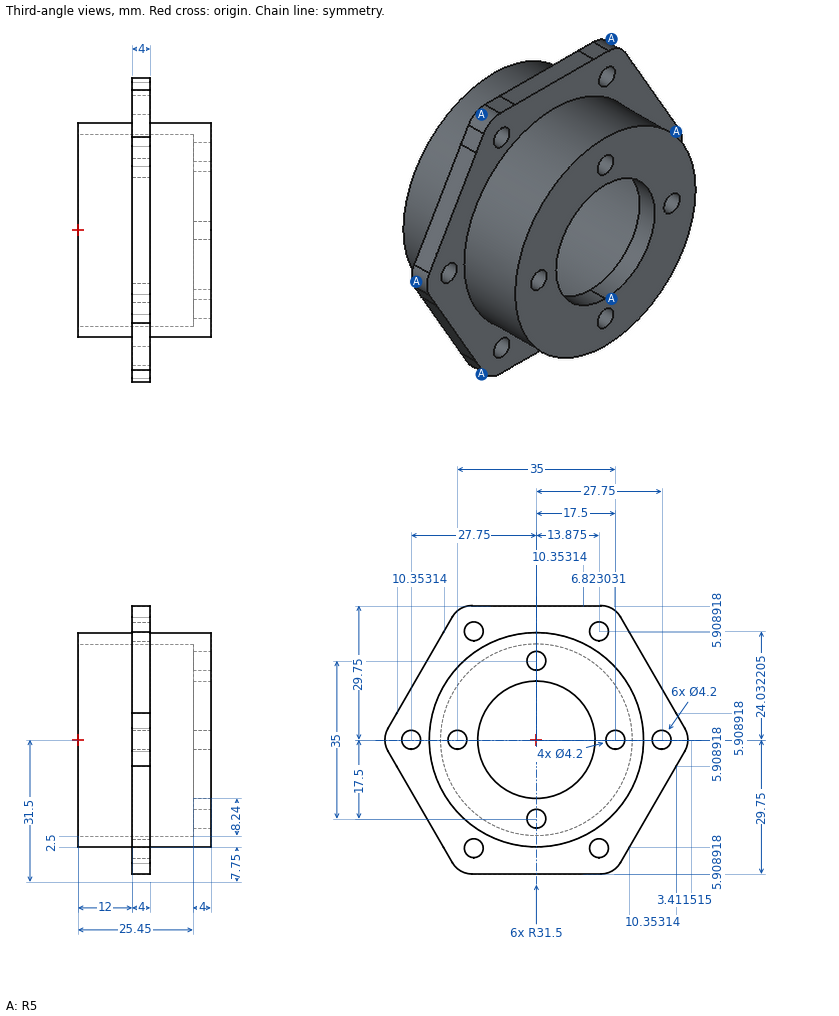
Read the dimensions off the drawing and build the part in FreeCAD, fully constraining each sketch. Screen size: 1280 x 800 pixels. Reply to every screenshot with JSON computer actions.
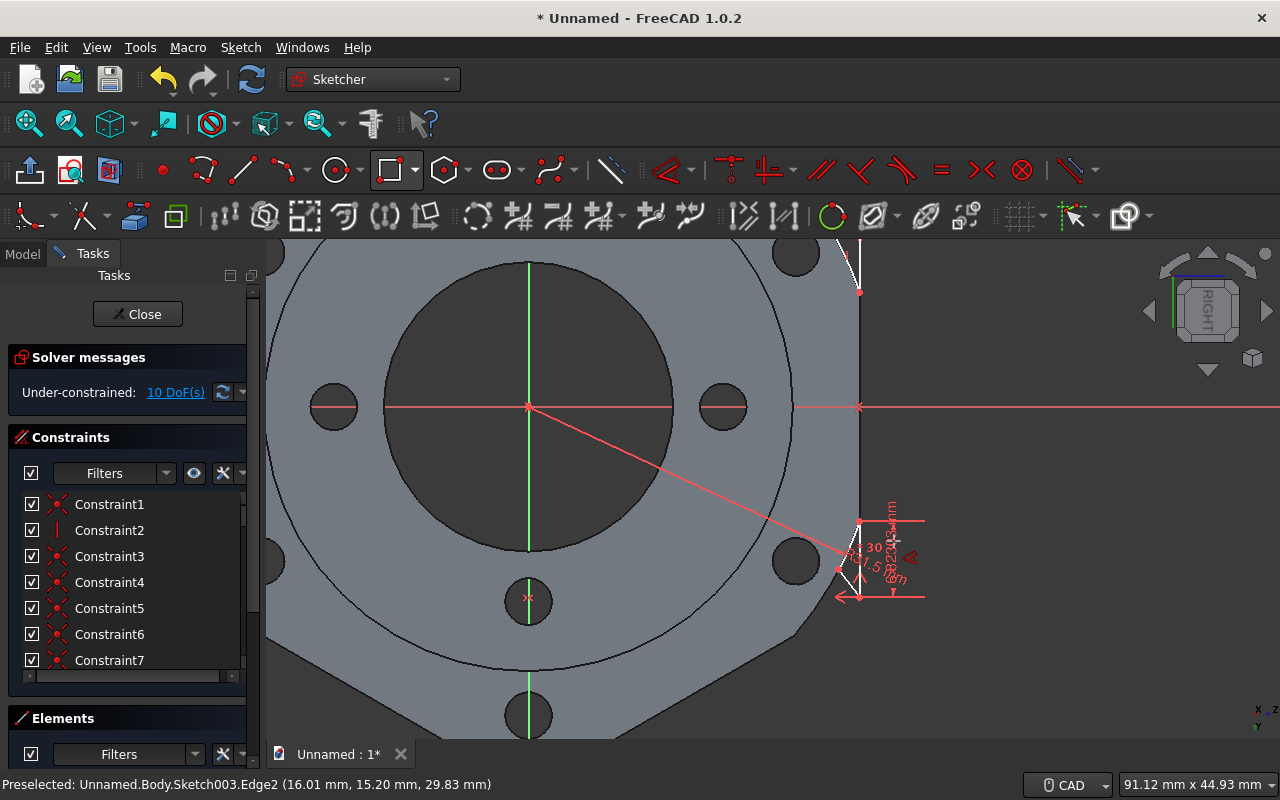
{"action": "left_click", "coordinate": [860, 521]}
{"action": "left_click", "coordinate": [894, 464]}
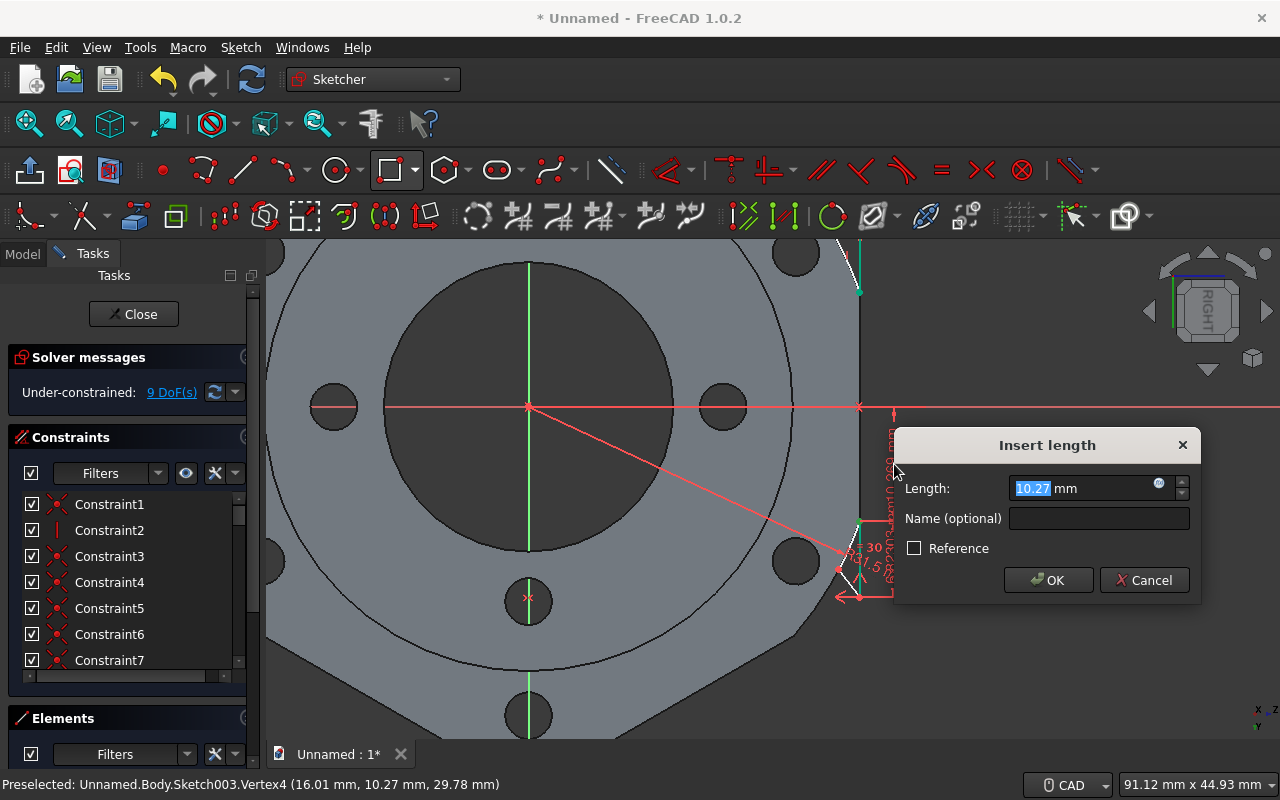
{"action": "type", "text": "10.35314"}
{"action": "key", "text": "Return"}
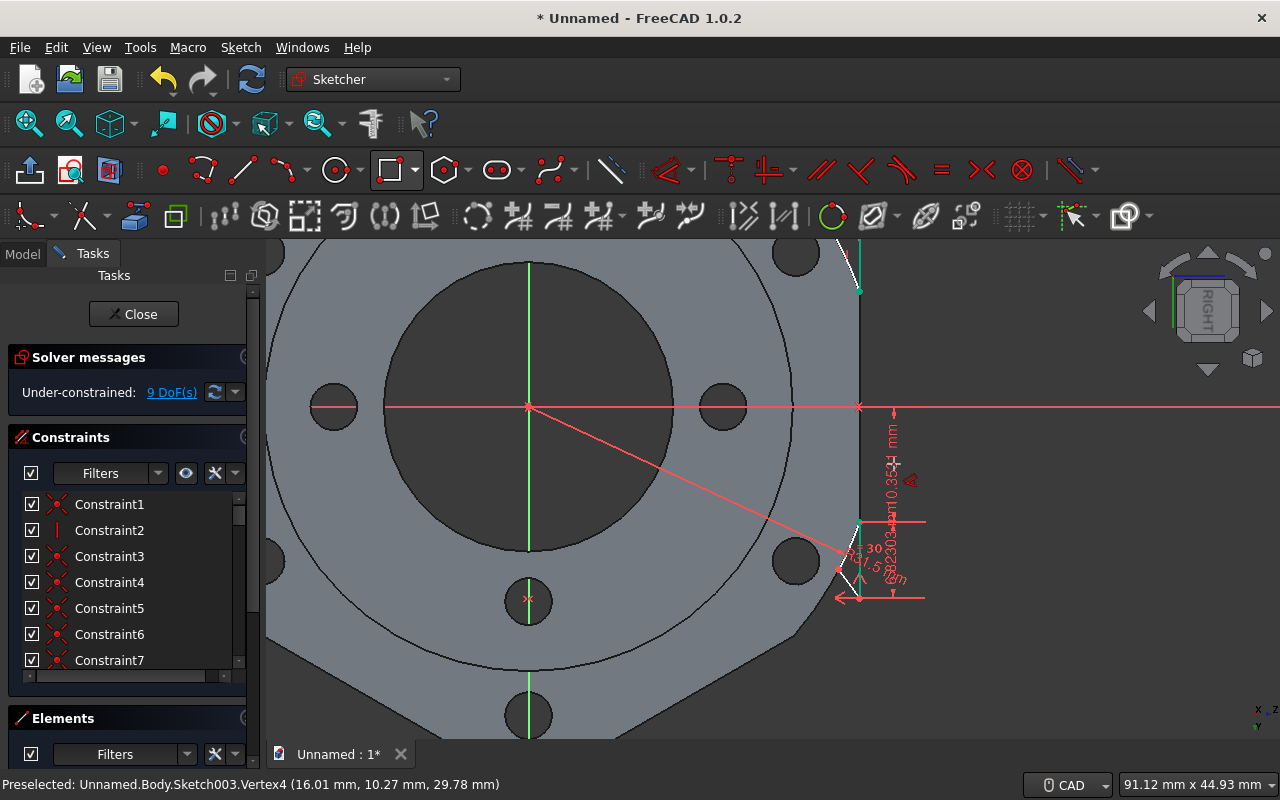
{"action": "scroll", "coordinate": [848, 556], "scroll_direction": "down", "scroll_amount": 4}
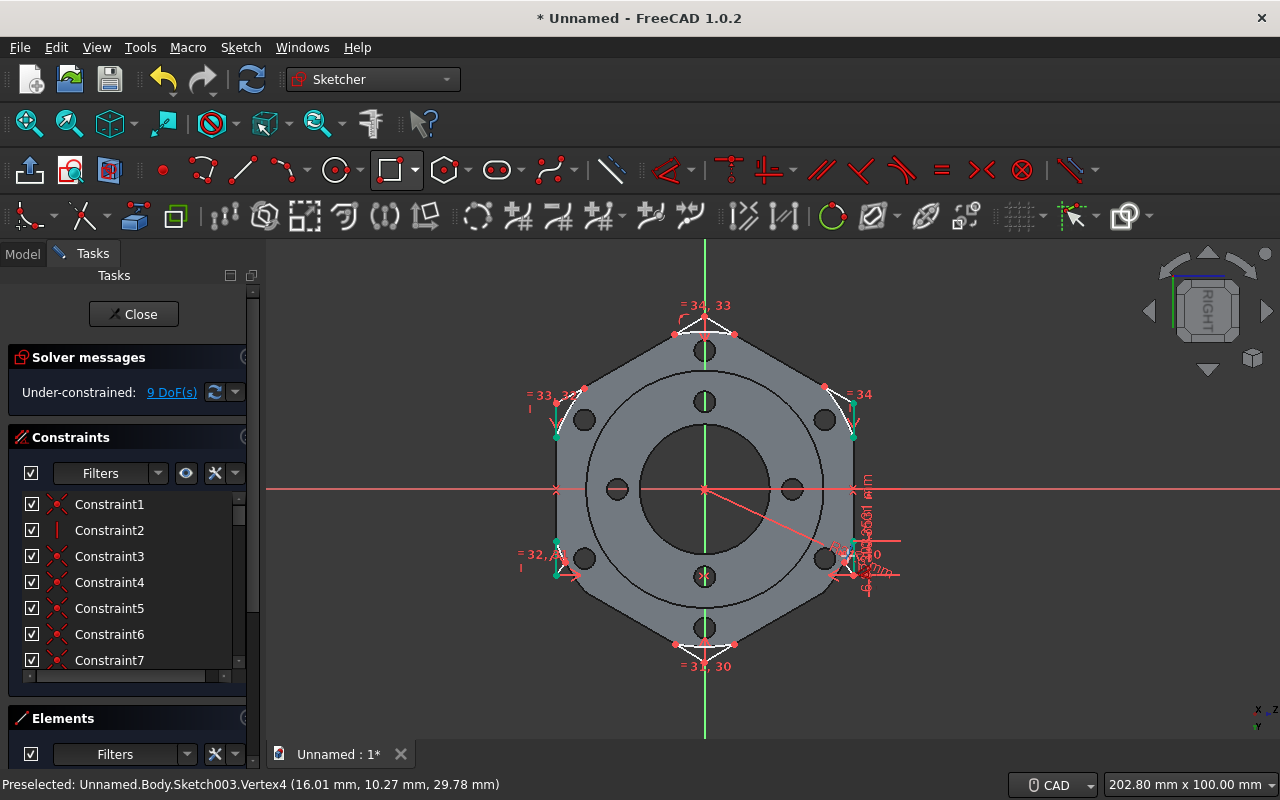
{"action": "scroll", "coordinate": [675, 644], "scroll_direction": "up", "scroll_amount": 2}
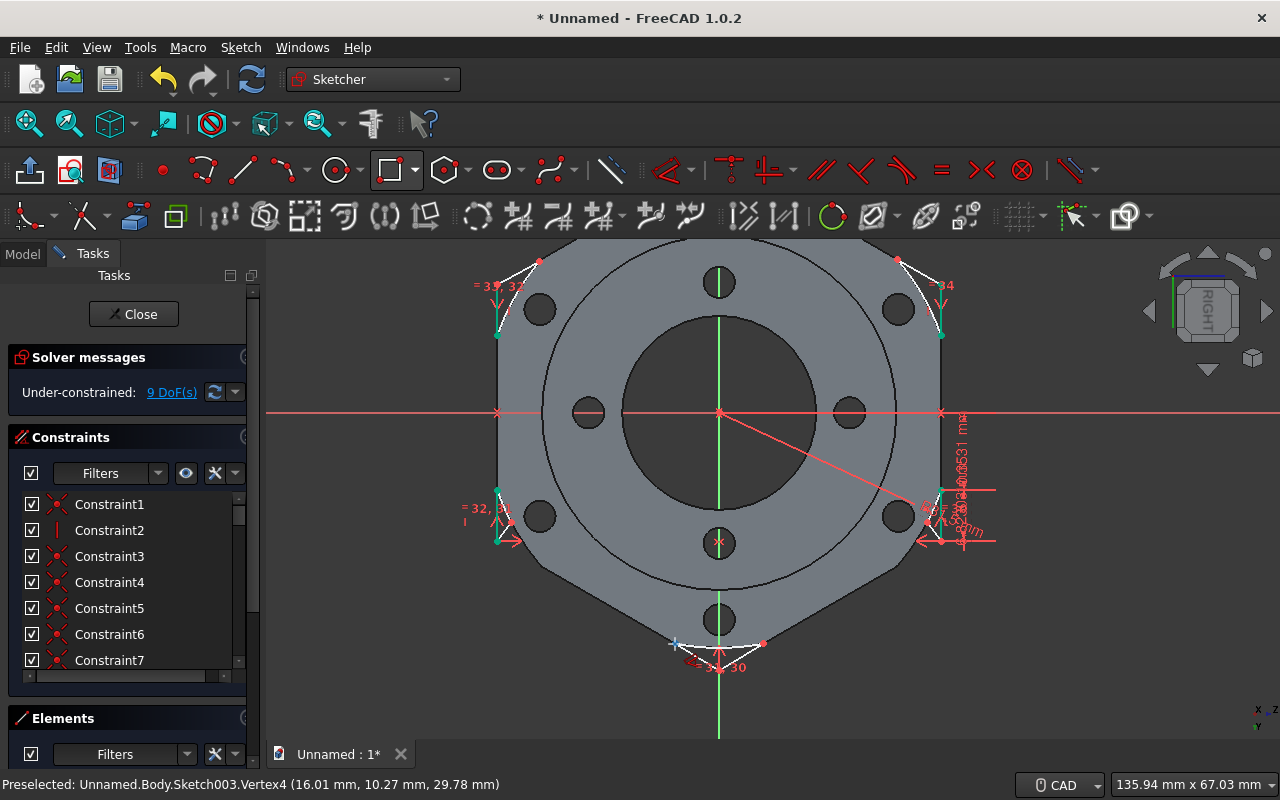
{"action": "left_click", "coordinate": [675, 644]}
{"action": "left_click", "coordinate": [697, 678]}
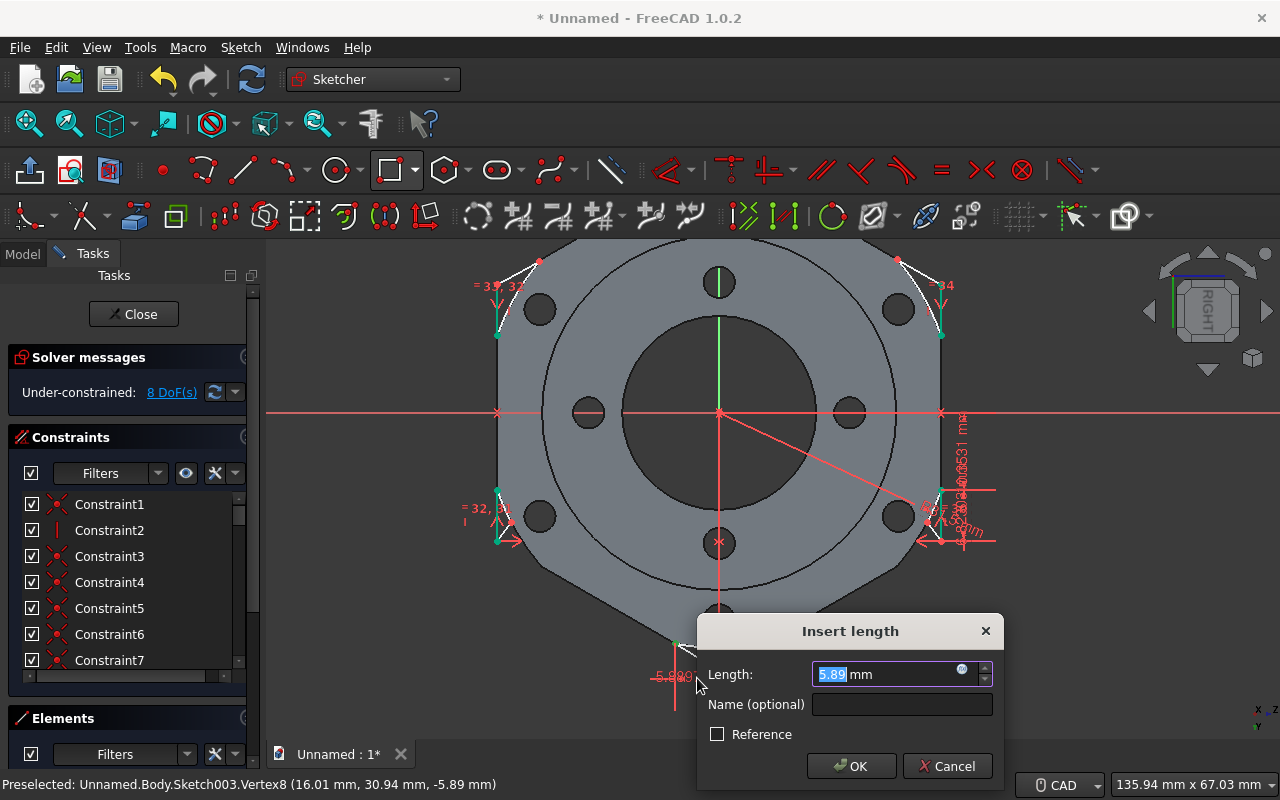
{"action": "type", "text": "5.908918"}
{"action": "key", "text": "Return"}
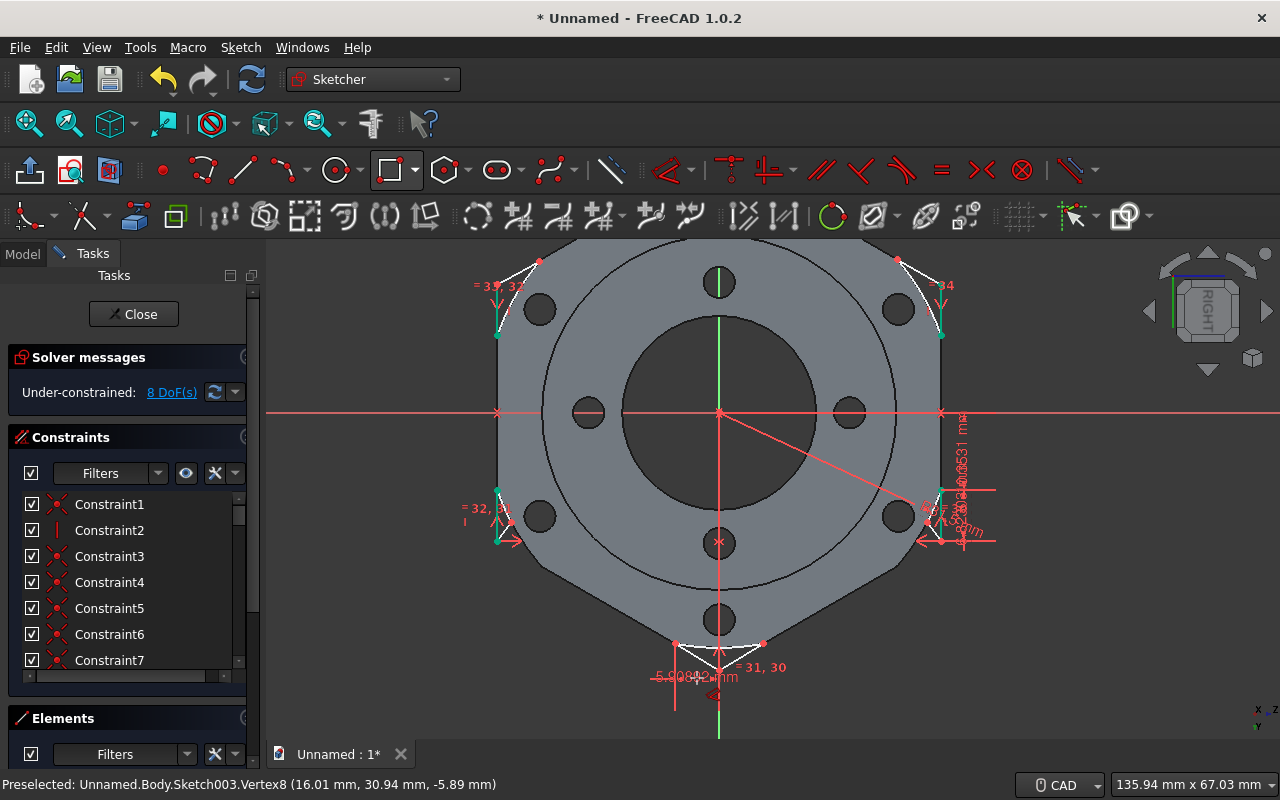
{"action": "left_click", "coordinate": [764, 644]}
{"action": "left_click", "coordinate": [741, 379]}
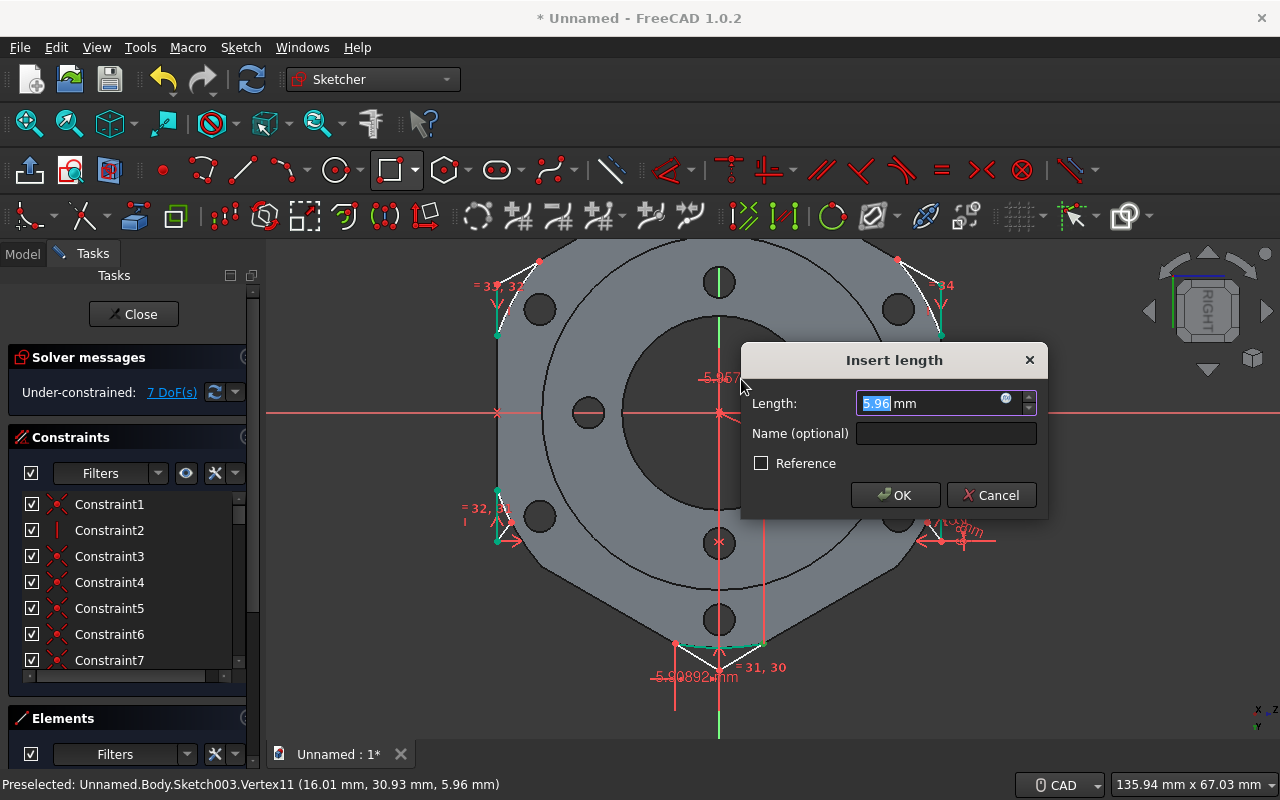
{"action": "type", "text": "5.908918"}
{"action": "key", "text": "Return"}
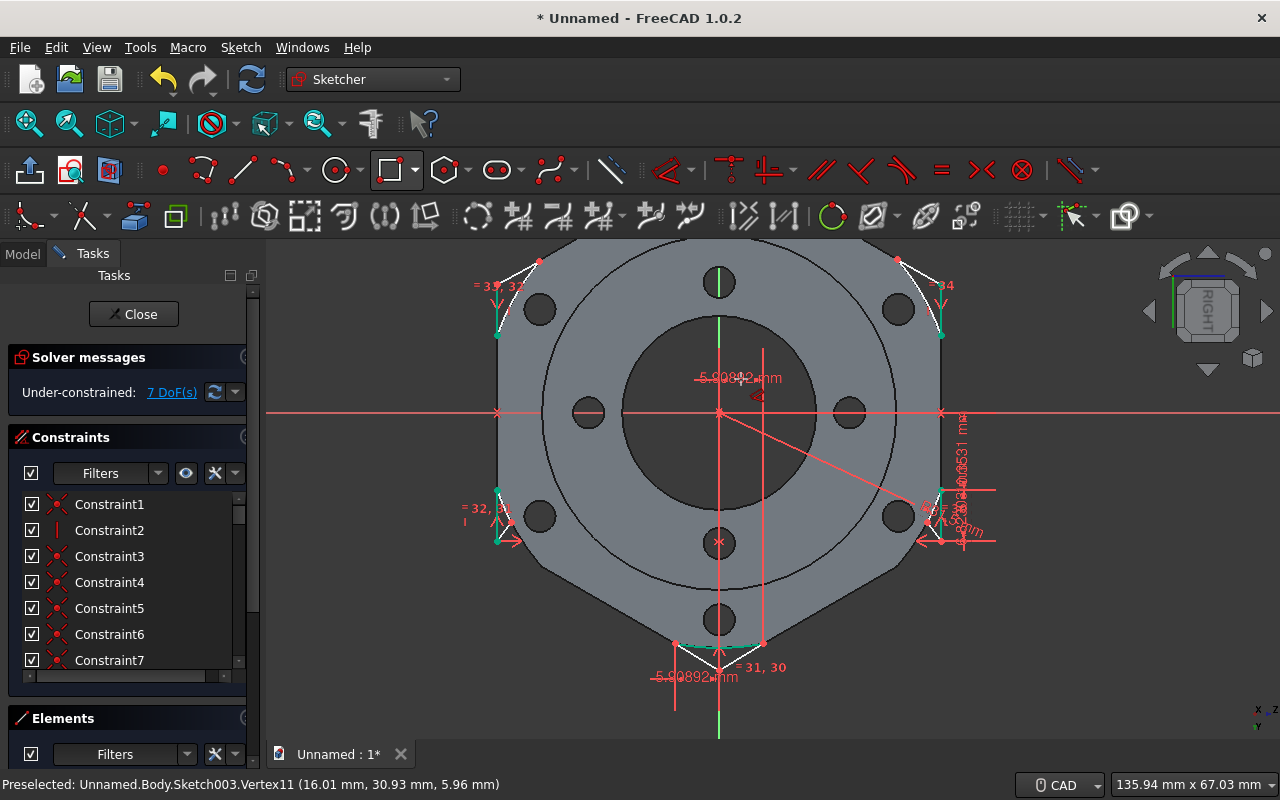
{"action": "scroll", "coordinate": [675, 644], "scroll_direction": "down", "scroll_amount": 2}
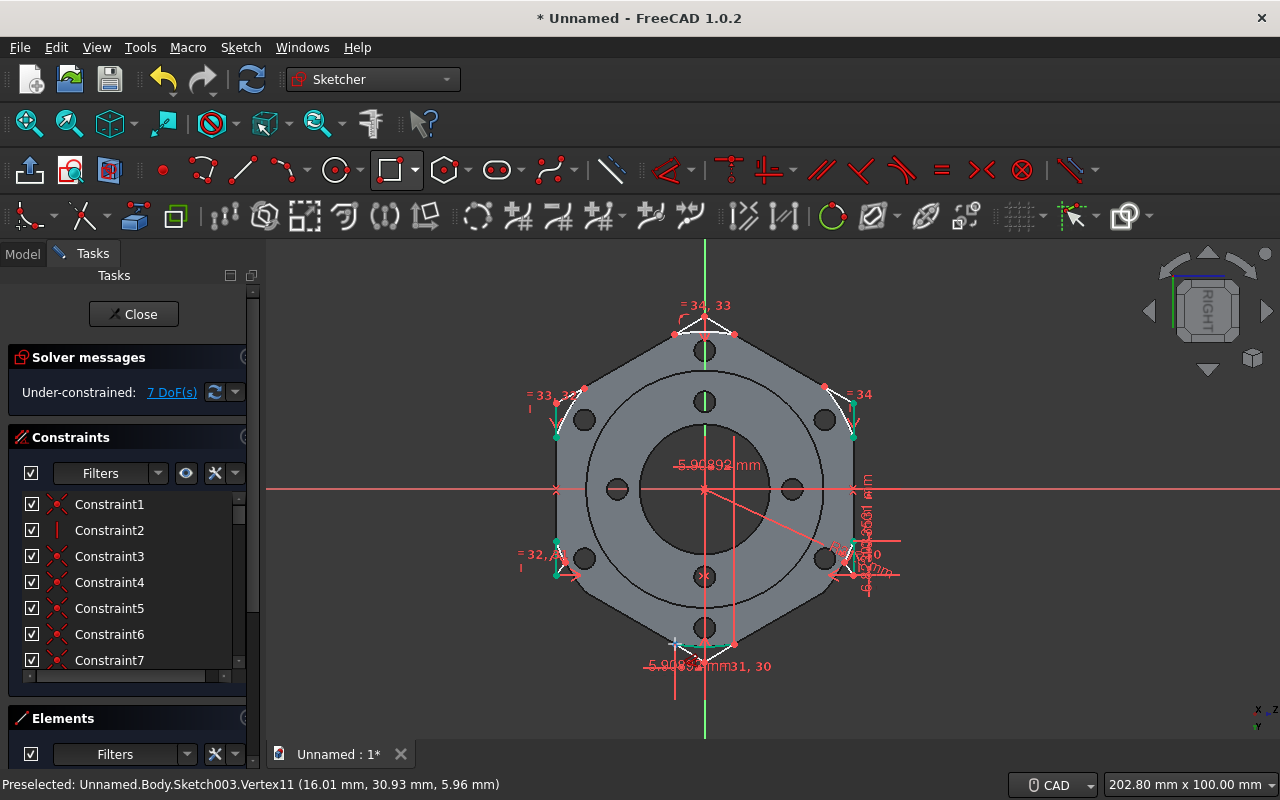
{"action": "scroll", "coordinate": [735, 335], "scroll_direction": "up", "scroll_amount": 2}